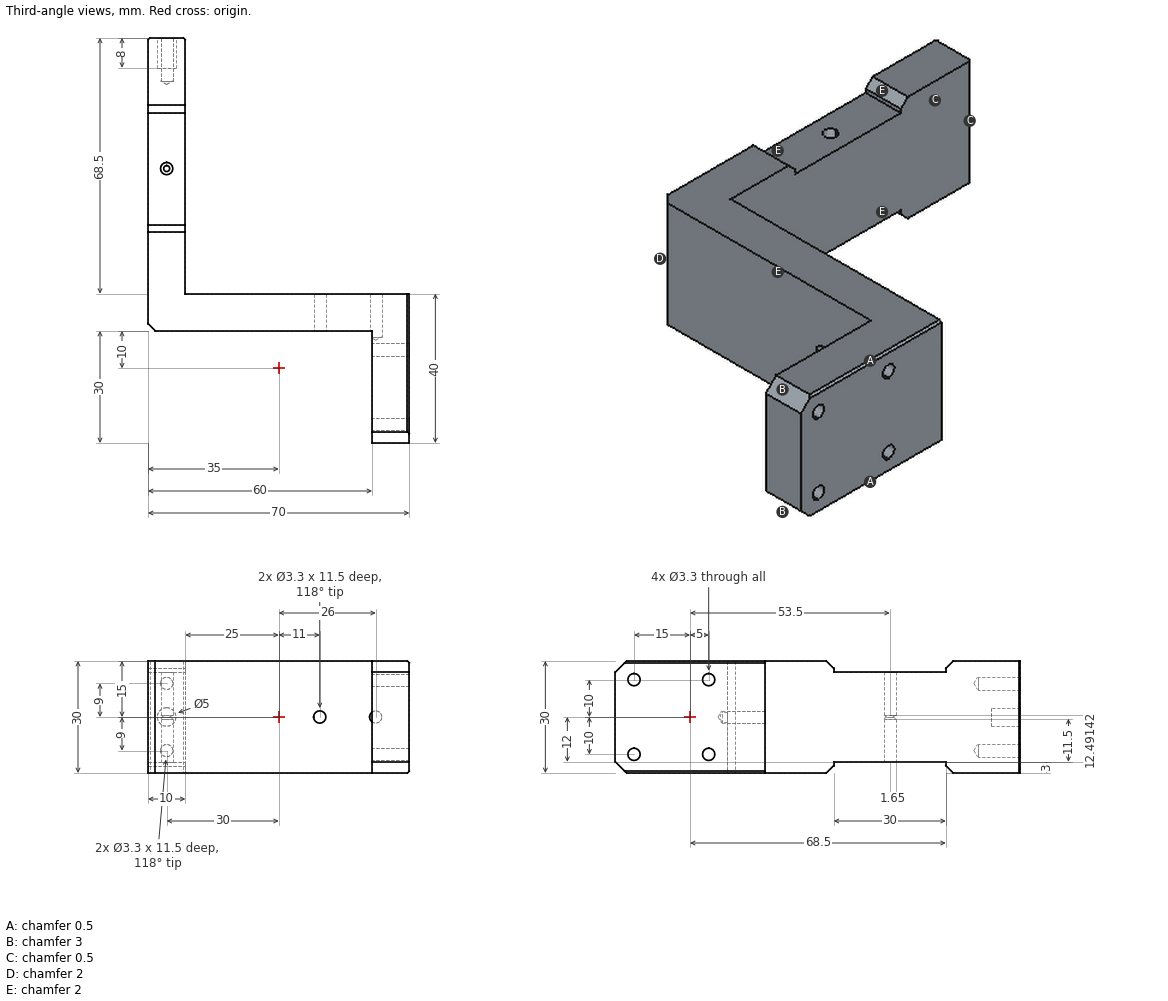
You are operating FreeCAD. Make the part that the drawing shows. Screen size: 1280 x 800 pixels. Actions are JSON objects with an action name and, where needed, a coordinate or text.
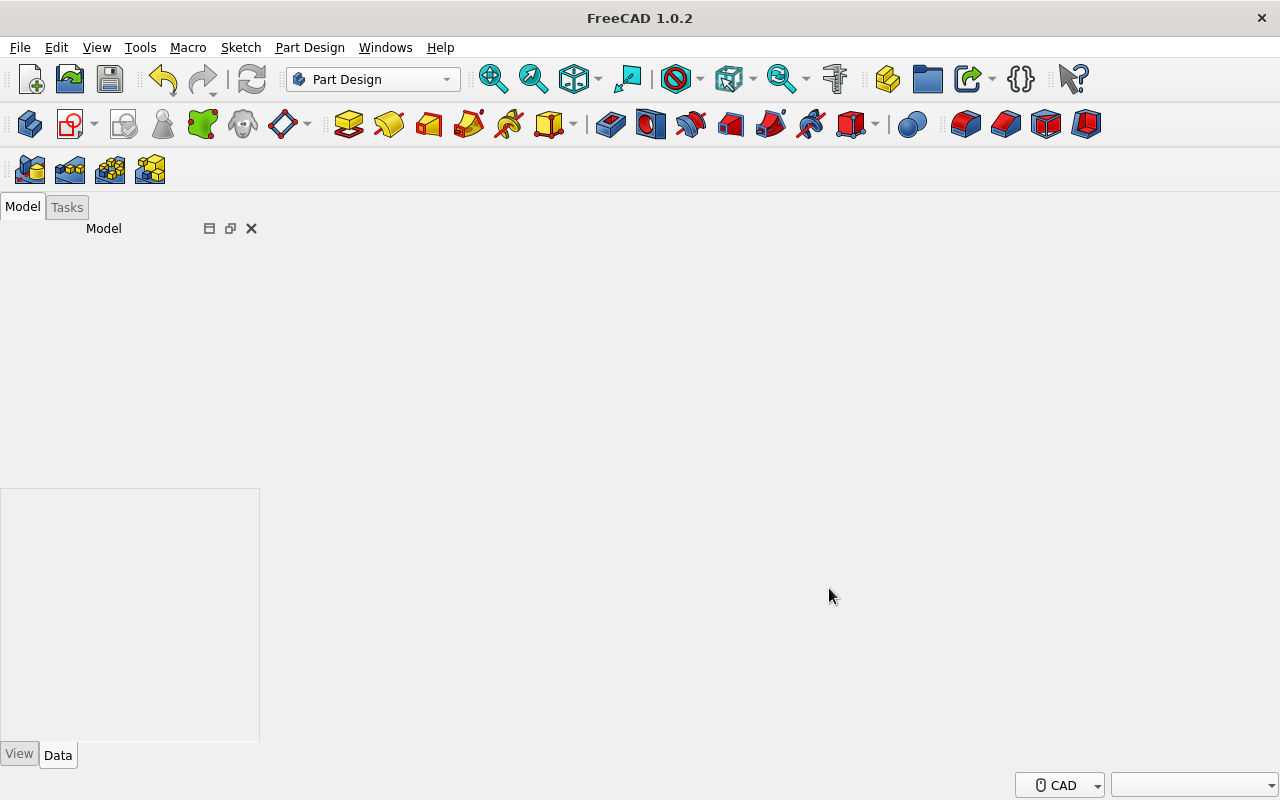
{"action": "key", "text": "ctrl+n"}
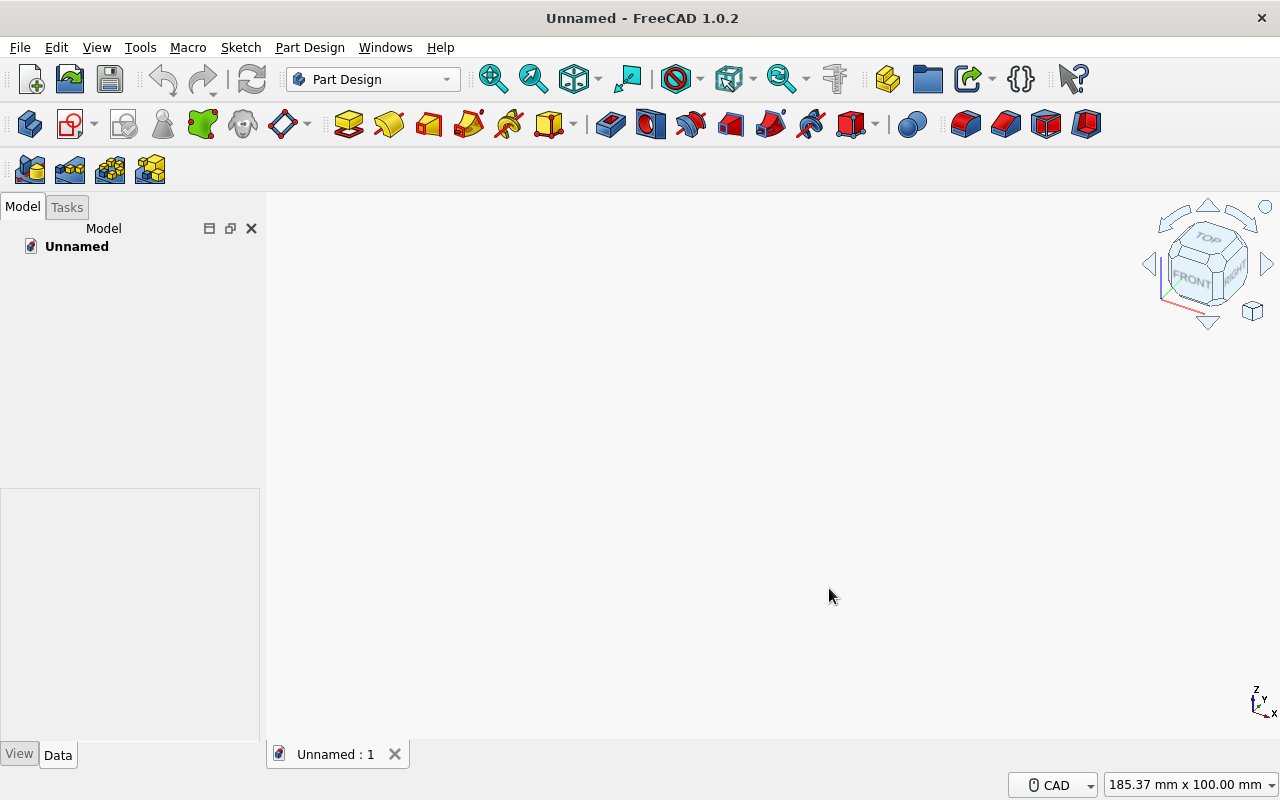
{"action": "left_click", "coordinate": [70, 124]}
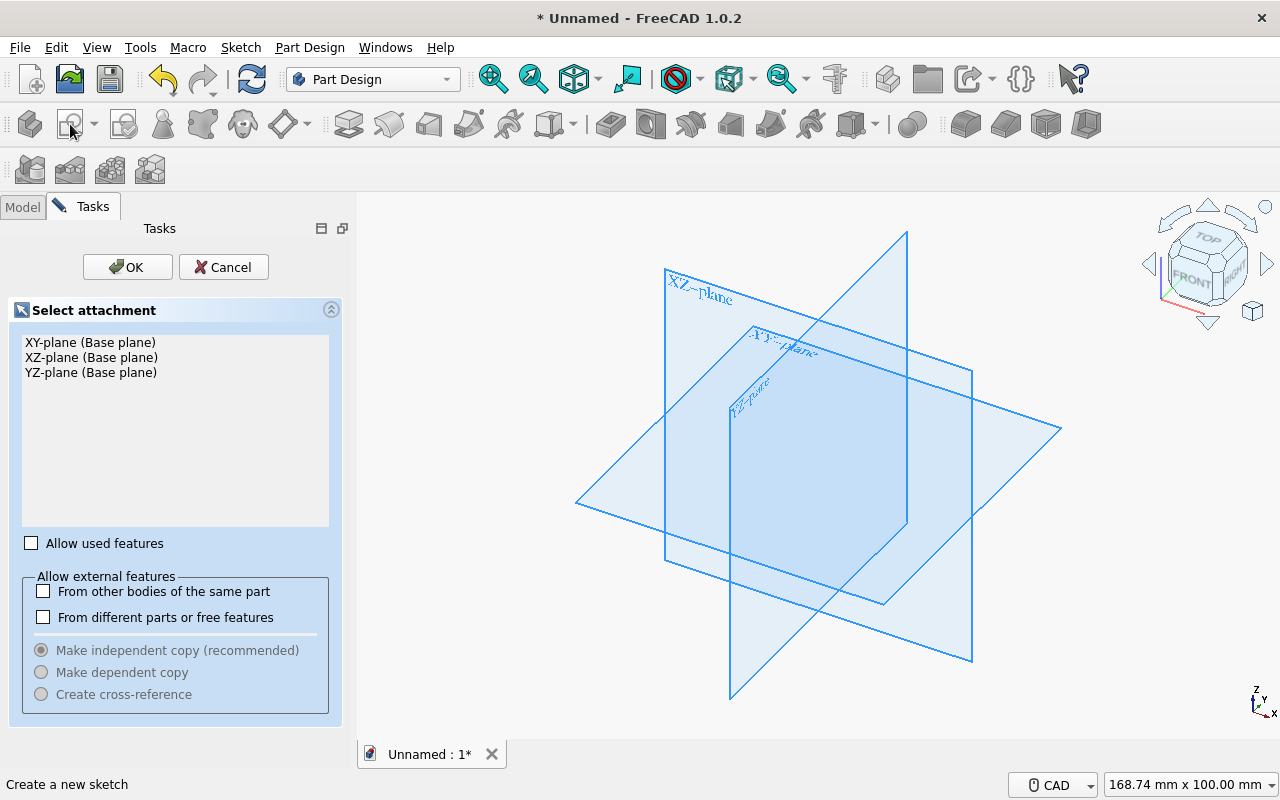
{"action": "left_click", "coordinate": [82, 342]}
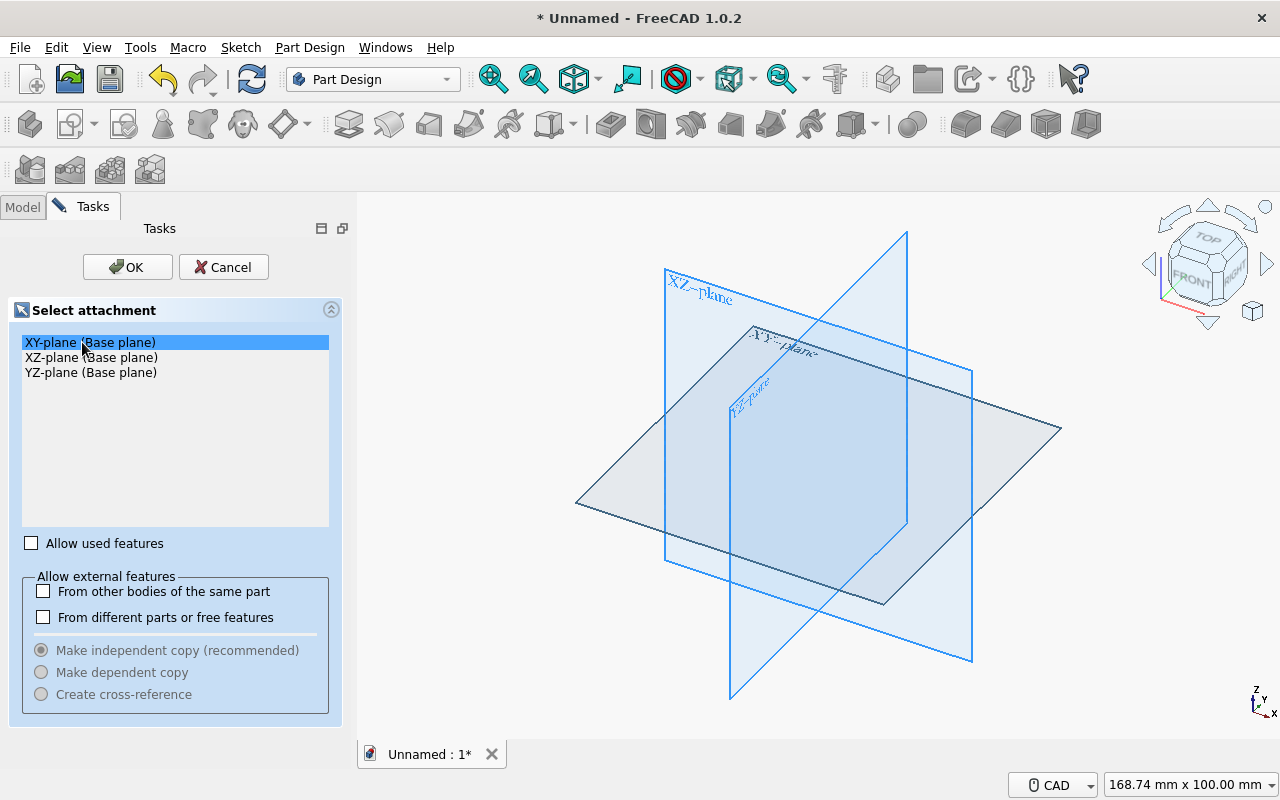
{"action": "left_click", "coordinate": [128, 267]}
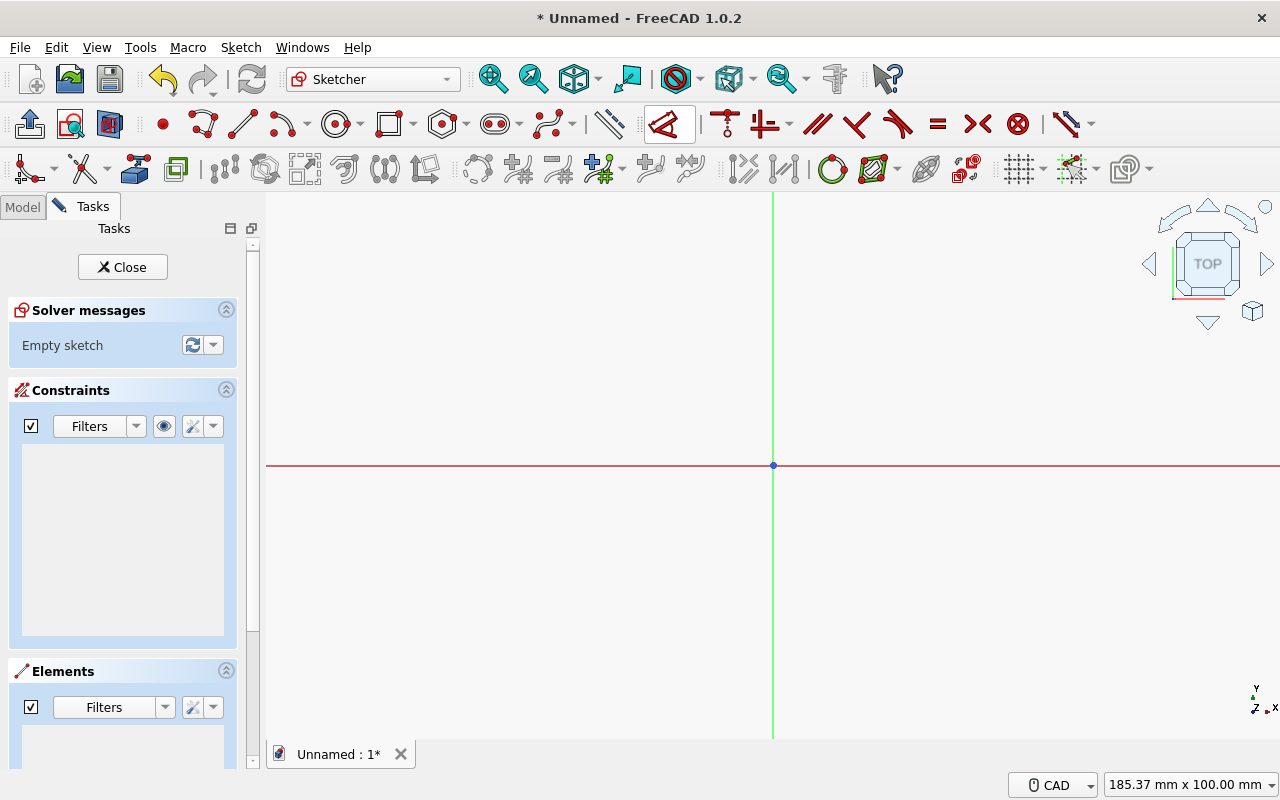
{"action": "scroll", "coordinate": [912, 466], "scroll_direction": "up", "scroll_amount": 2}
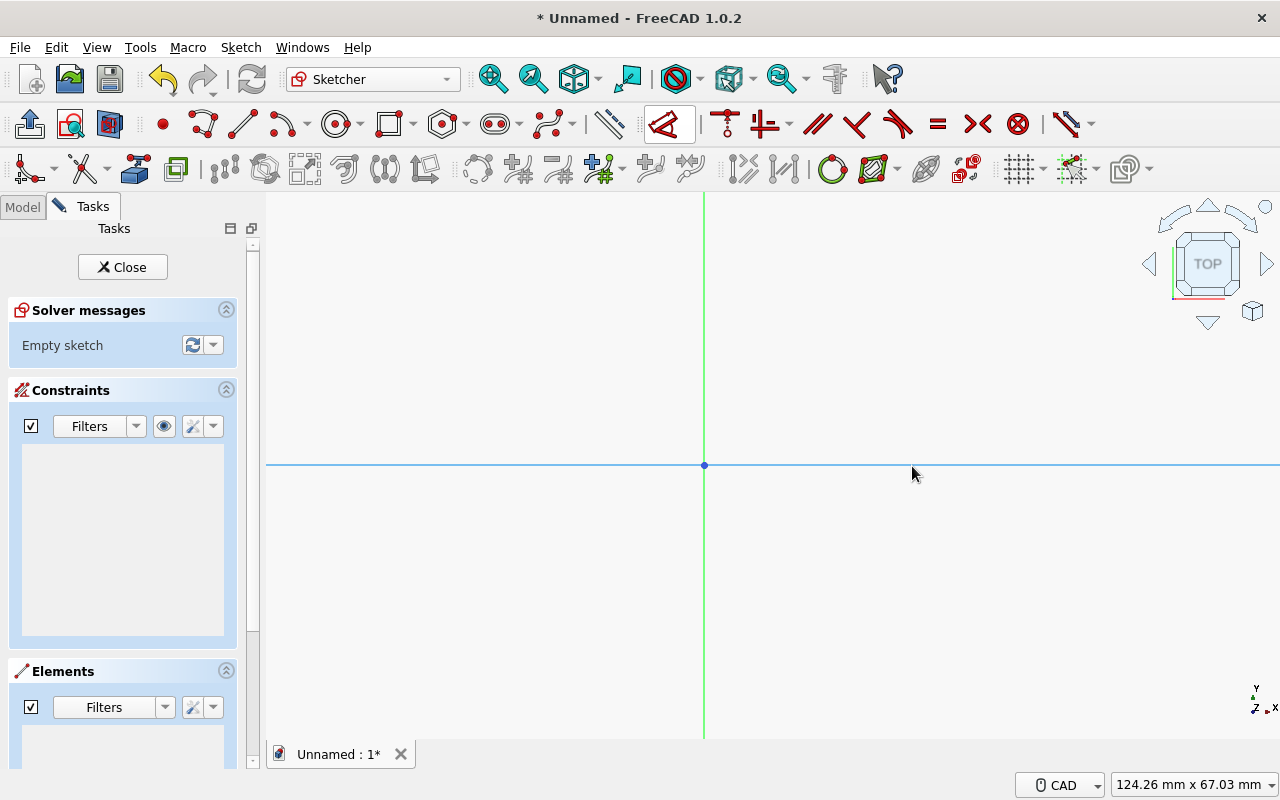
{"action": "key", "text": "g v"}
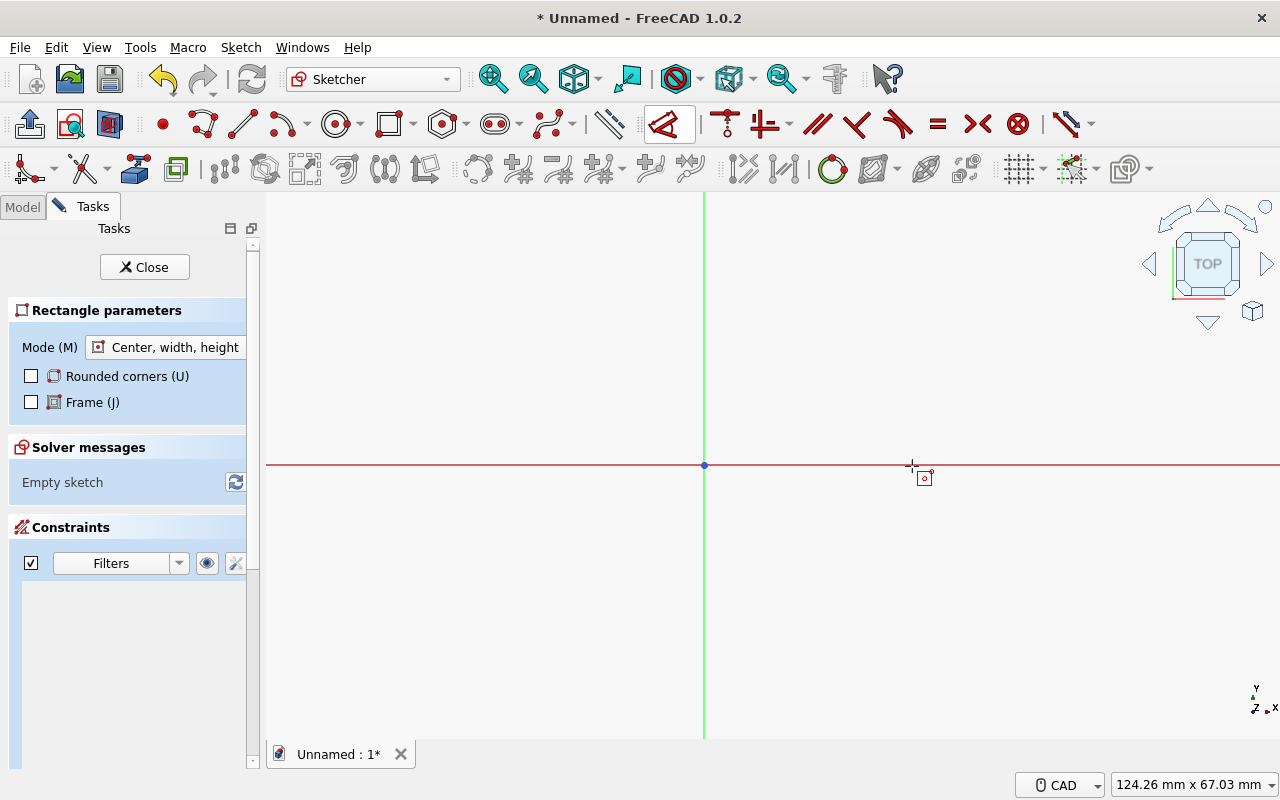
{"action": "left_click", "coordinate": [704, 465]}
{"action": "left_click", "coordinate": [990, 302]}
{"action": "key", "text": "Escape"}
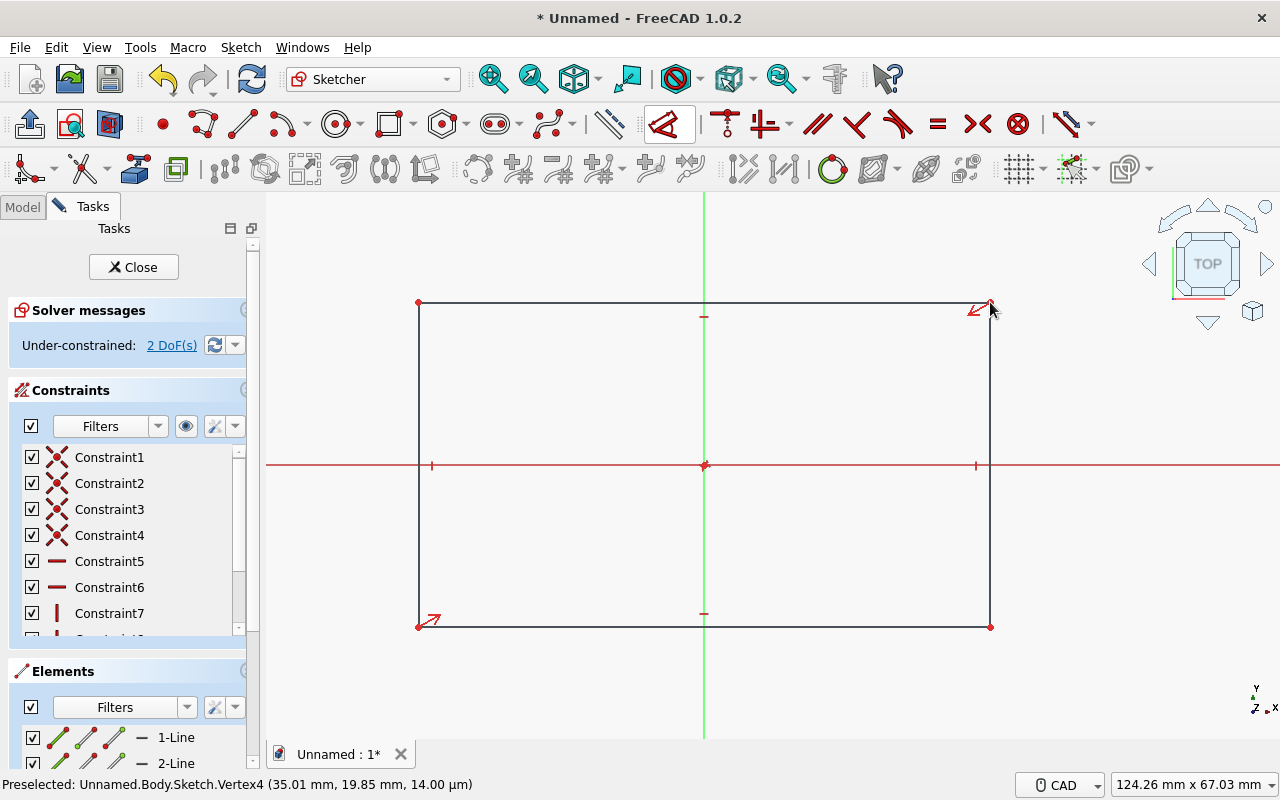
{"action": "left_click", "coordinate": [590, 627]}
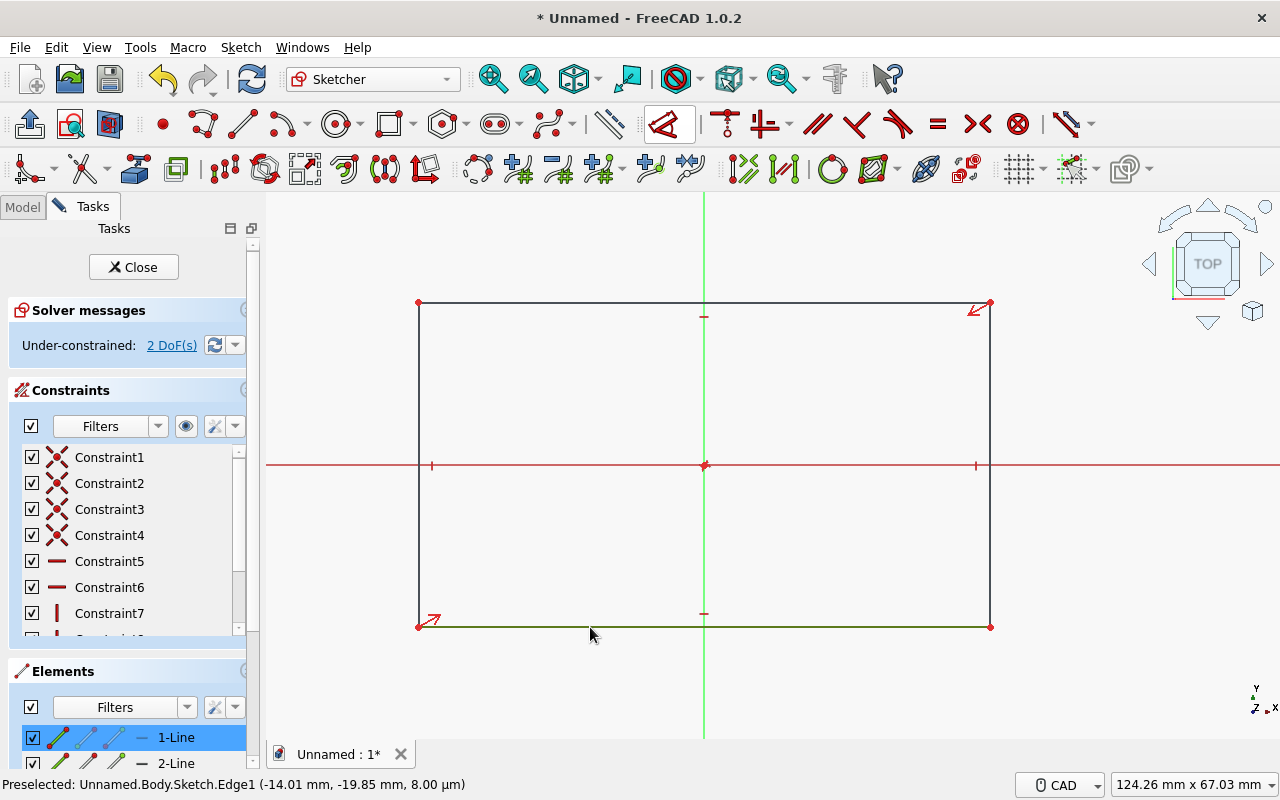
{"action": "key", "text": "l"}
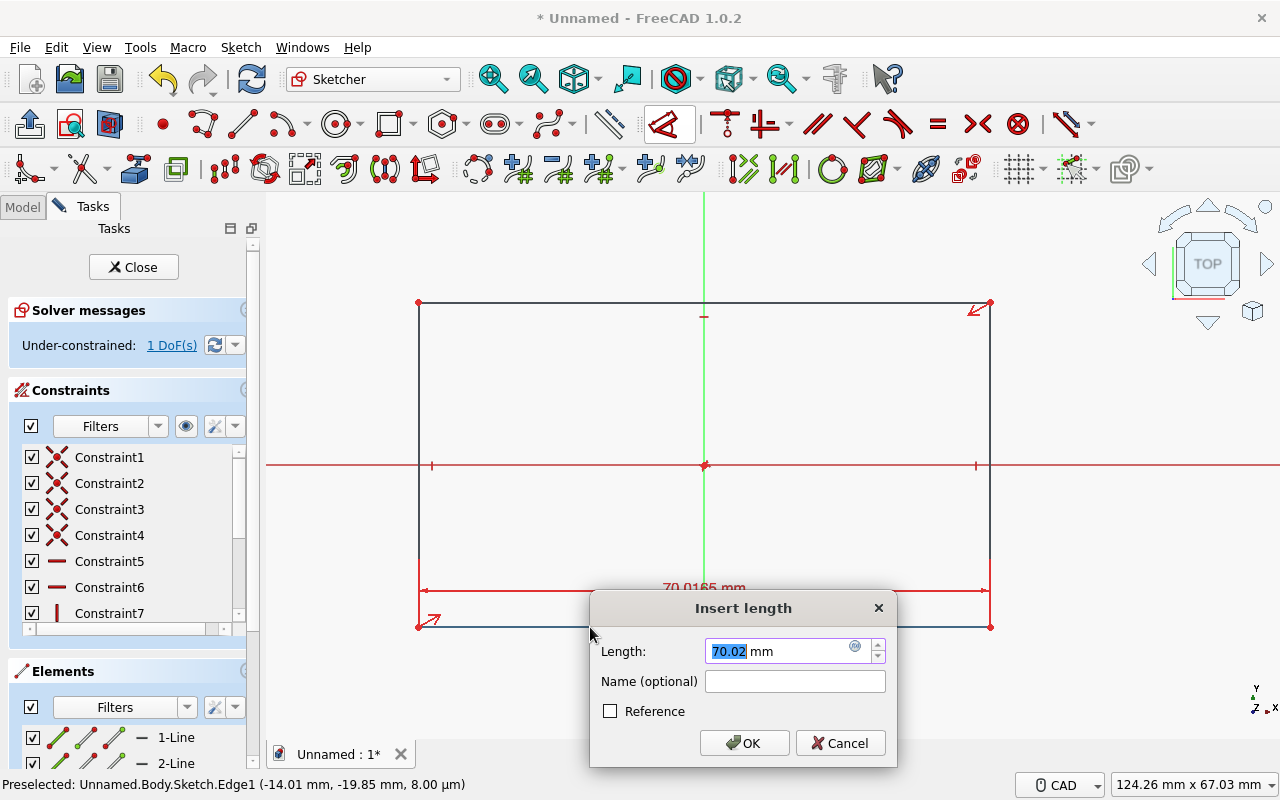
{"action": "type", "text": "70"}
{"action": "key", "text": "Return"}